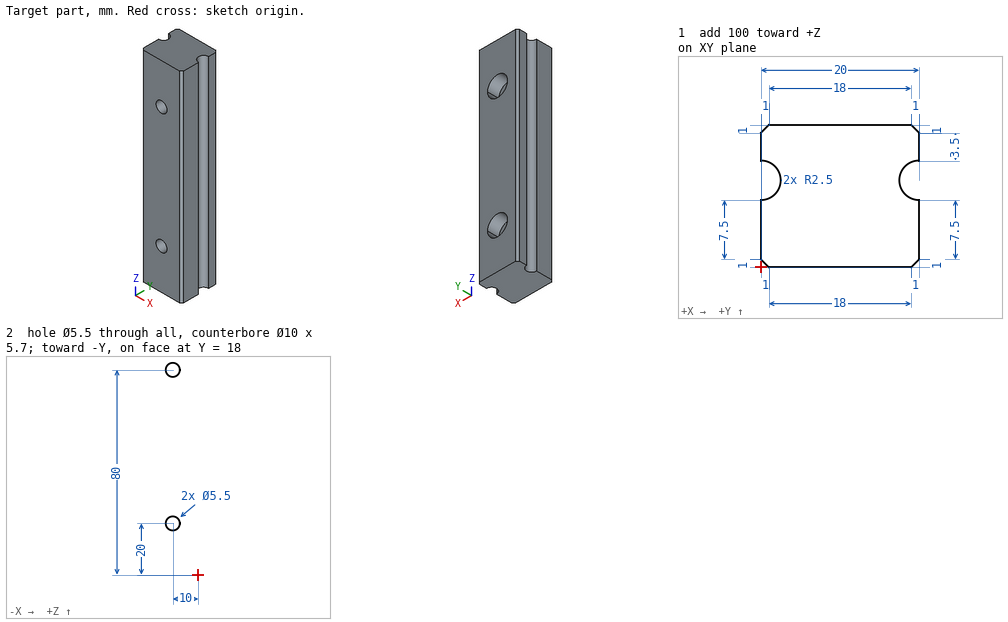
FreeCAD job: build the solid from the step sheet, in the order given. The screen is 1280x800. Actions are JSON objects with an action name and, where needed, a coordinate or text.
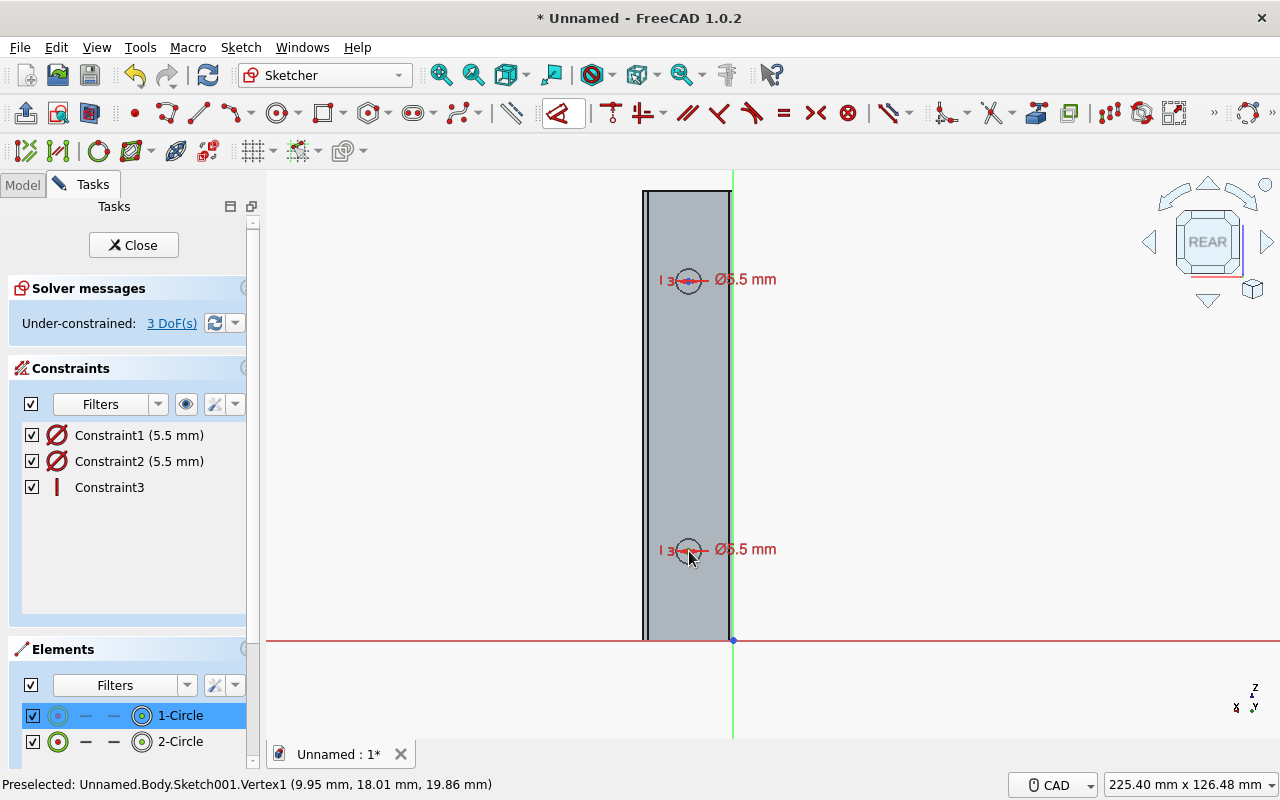
{"action": "left_click", "coordinate": [580, 114]}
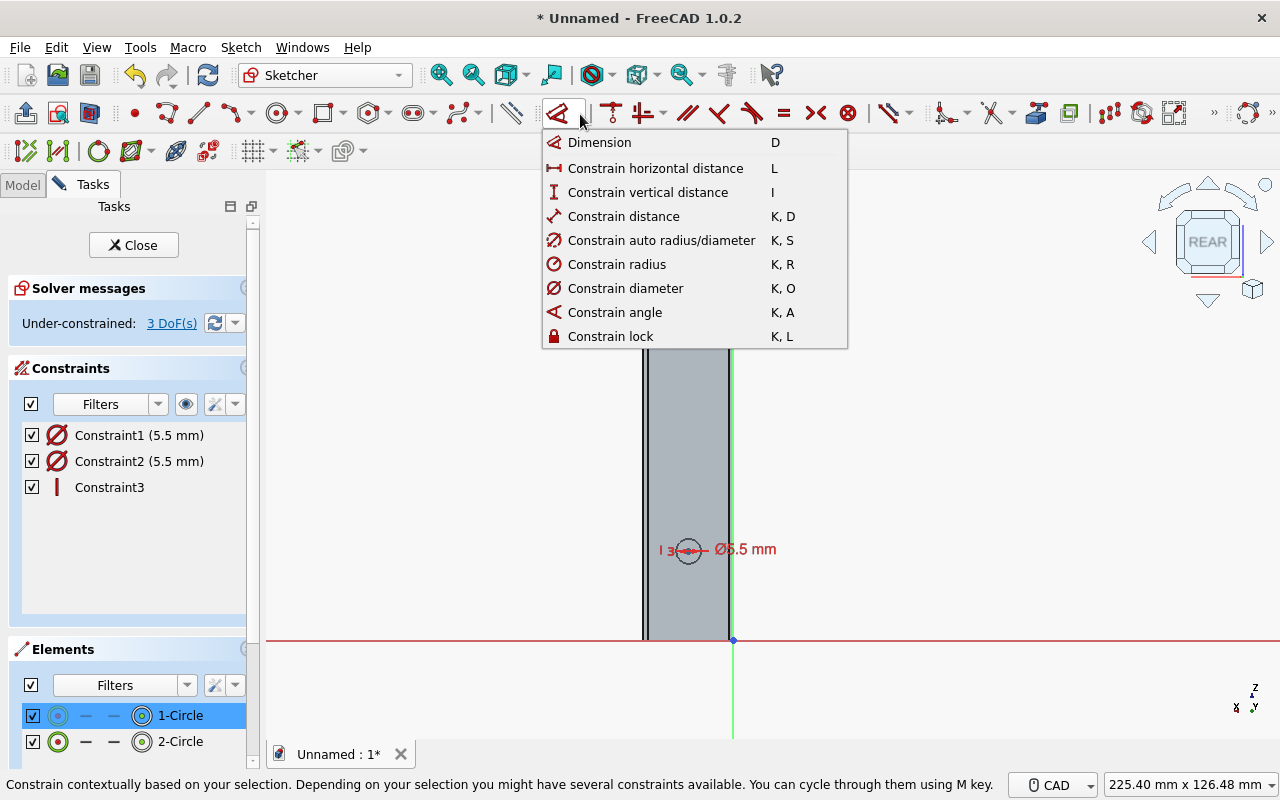
{"action": "left_click", "coordinate": [695, 168]}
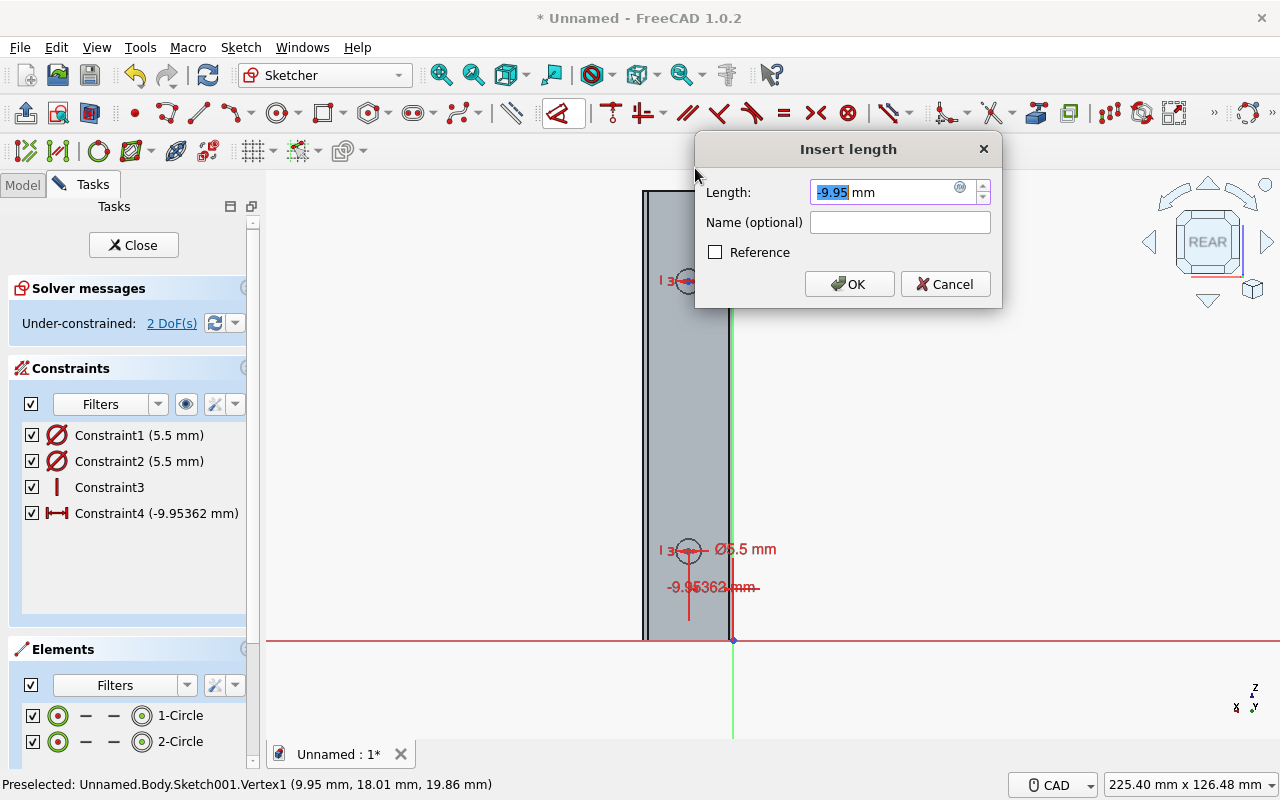
{"action": "type", "text": "-10"}
{"action": "key", "text": "Return"}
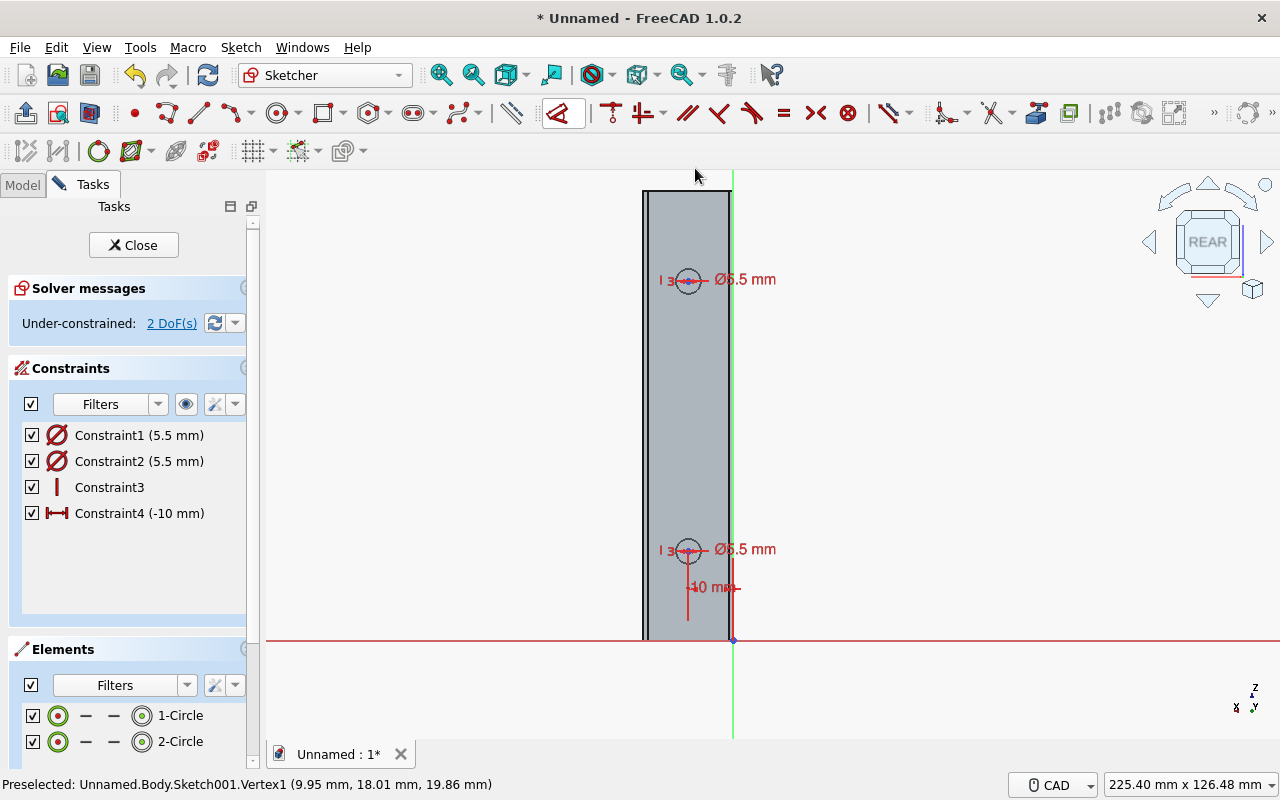
{"action": "left_click", "coordinate": [688, 551]}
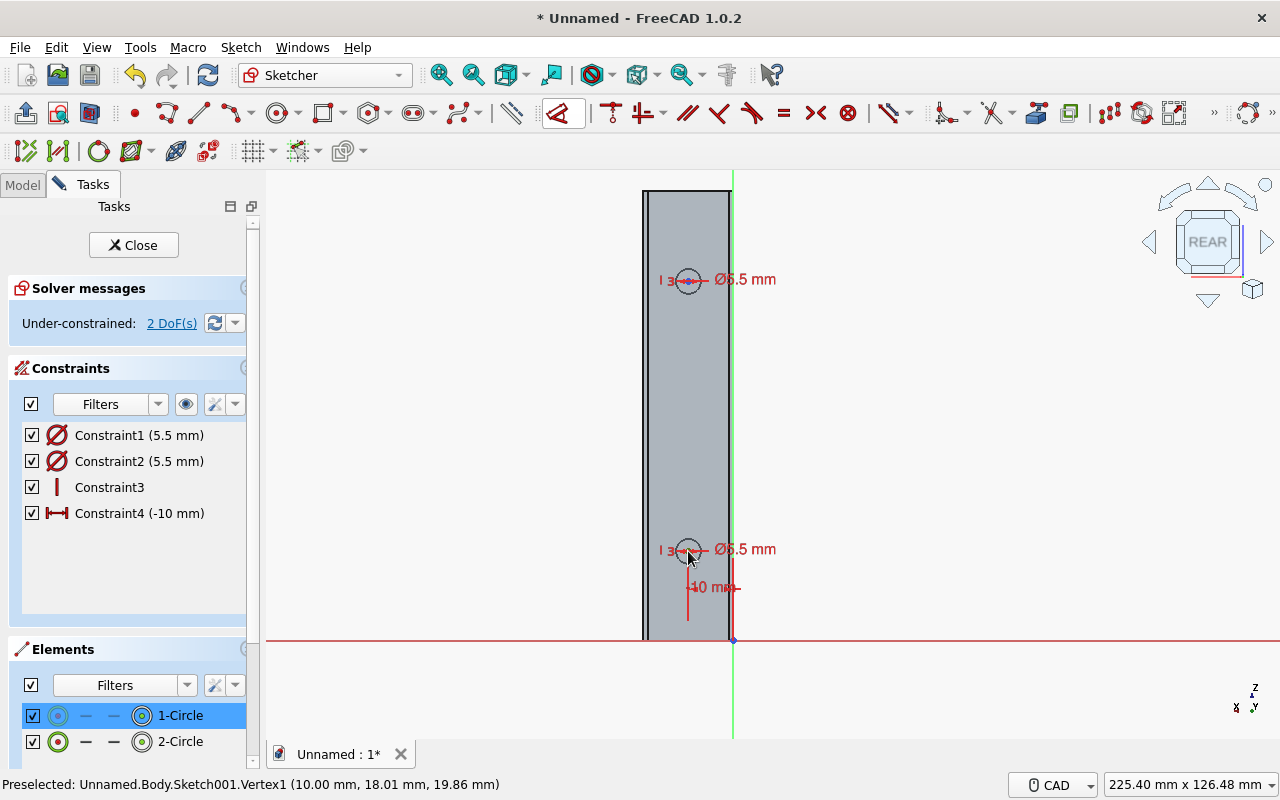
{"action": "key", "text": "i"}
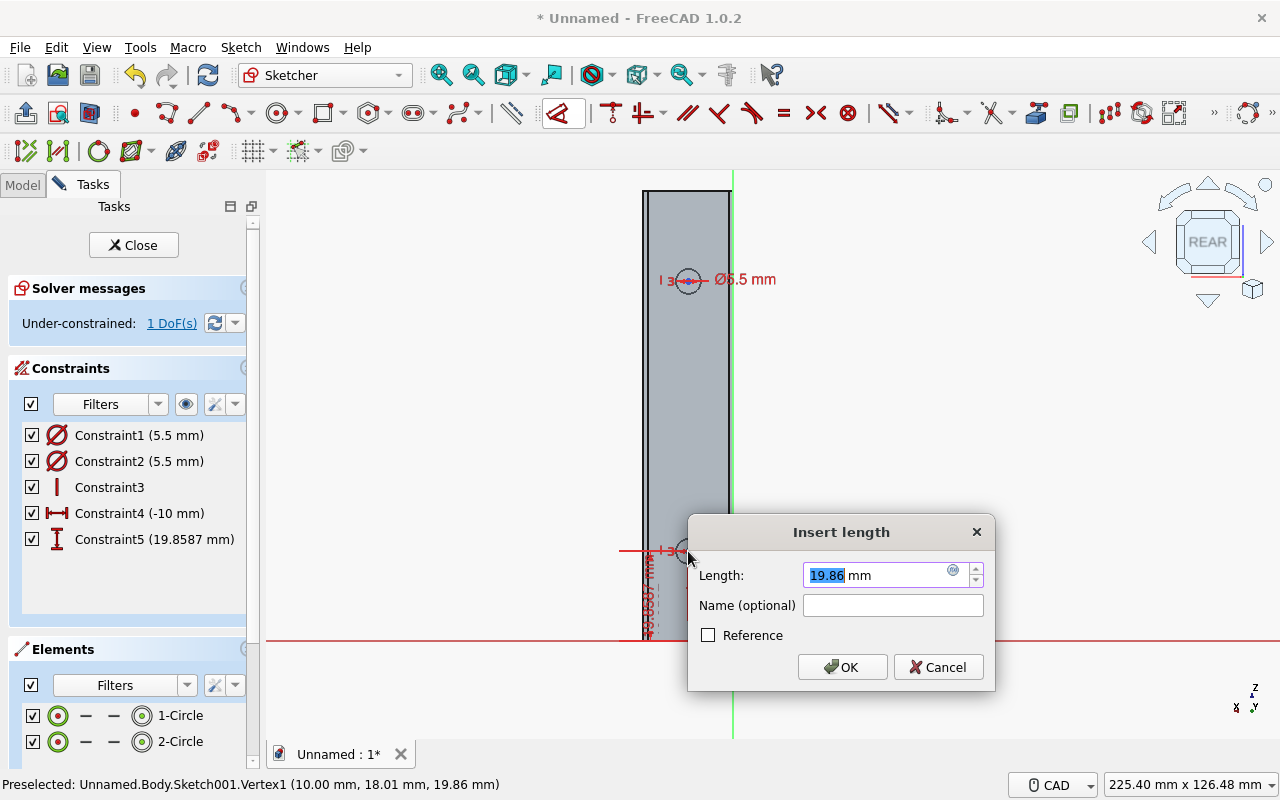
{"action": "type", "text": "20"}
{"action": "key", "text": "Return"}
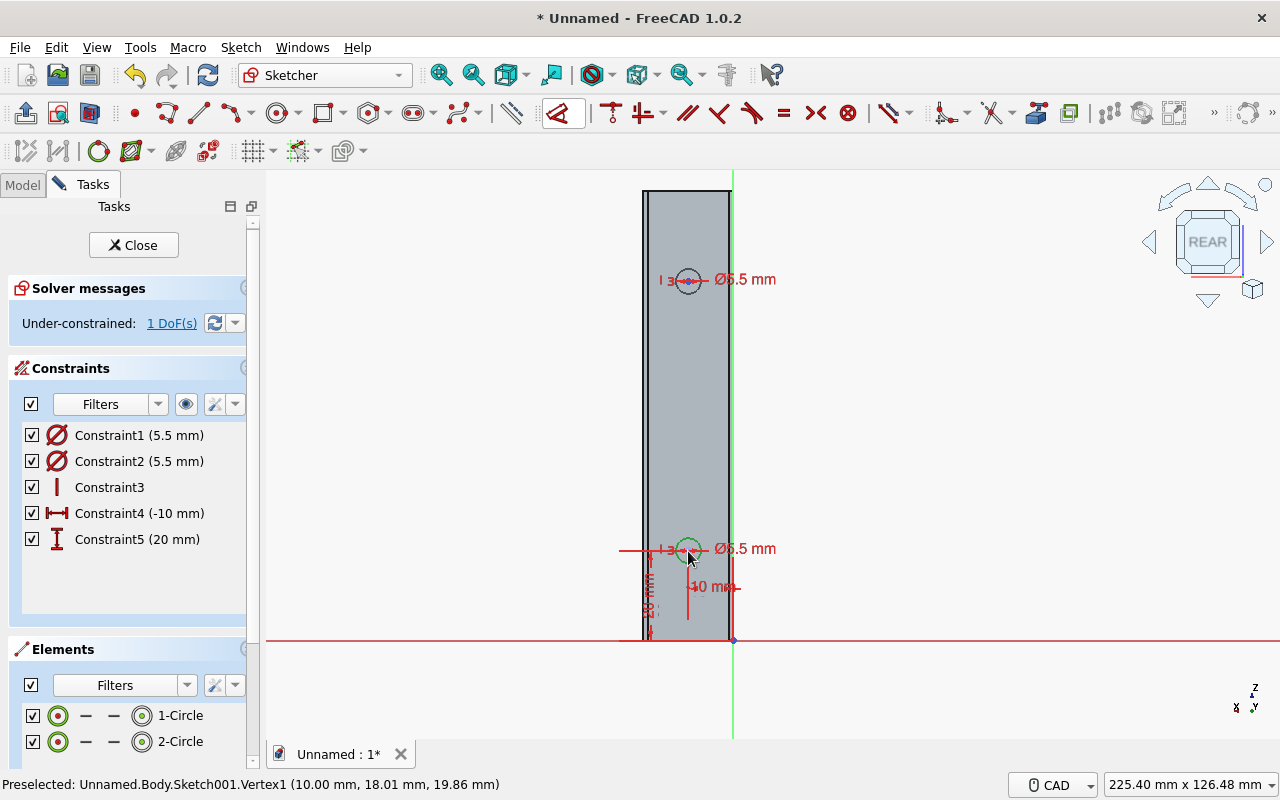
{"action": "left_click", "coordinate": [688, 281]}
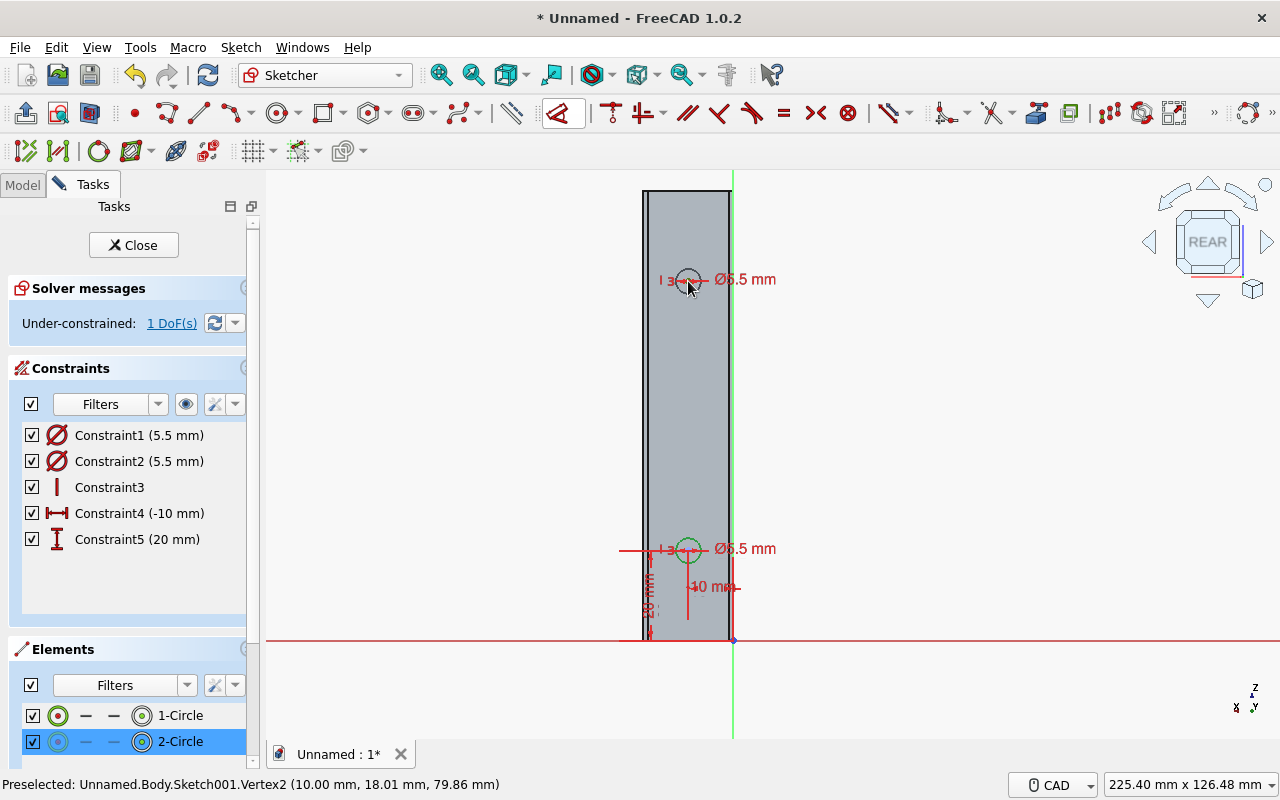
{"action": "key", "text": "i"}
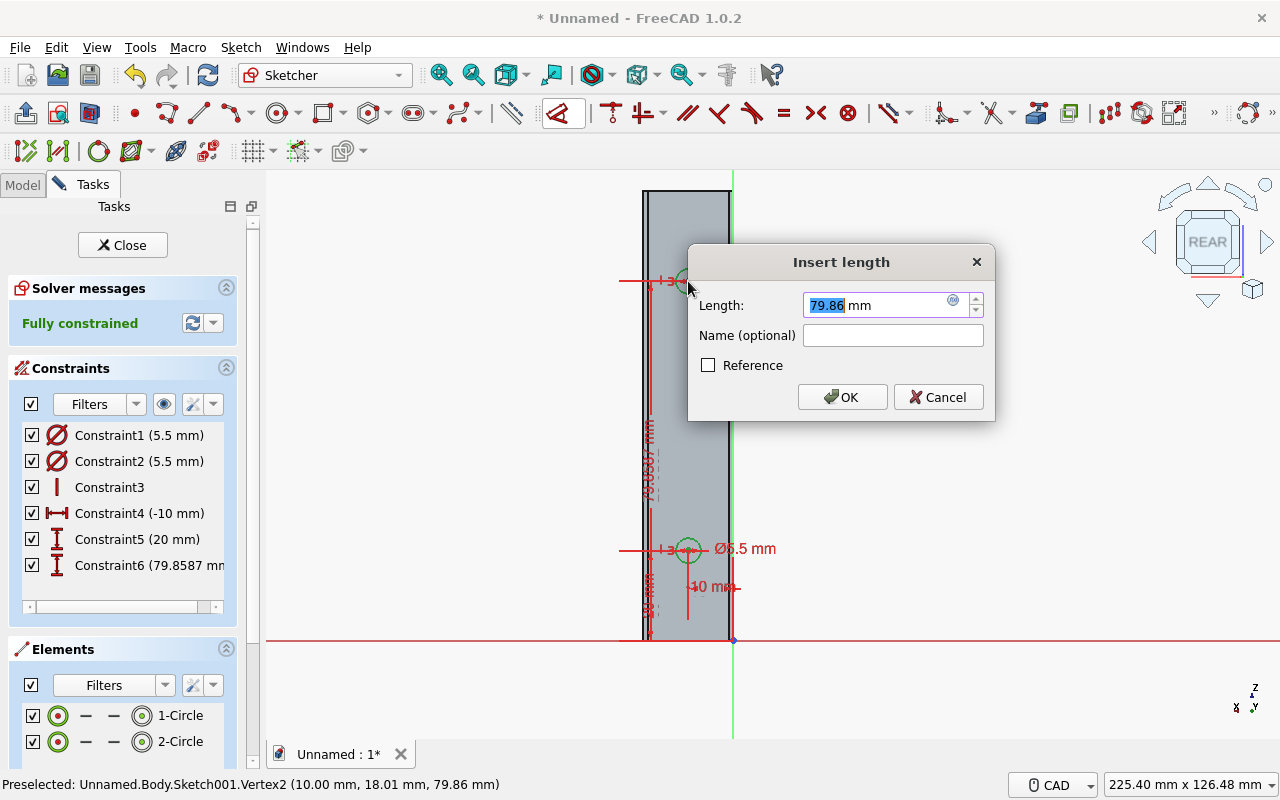
{"action": "type", "text": "80"}
{"action": "key", "text": "Return"}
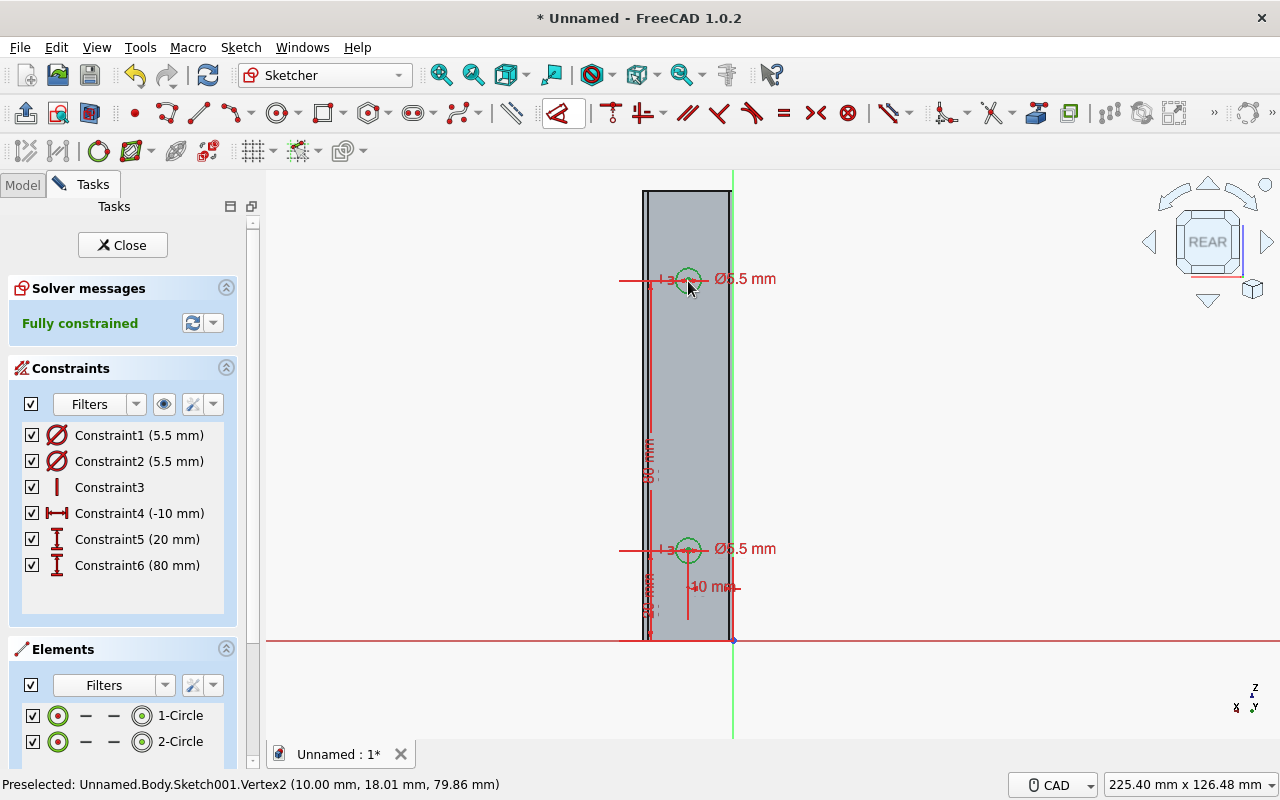
{"action": "left_click", "coordinate": [123, 245]}